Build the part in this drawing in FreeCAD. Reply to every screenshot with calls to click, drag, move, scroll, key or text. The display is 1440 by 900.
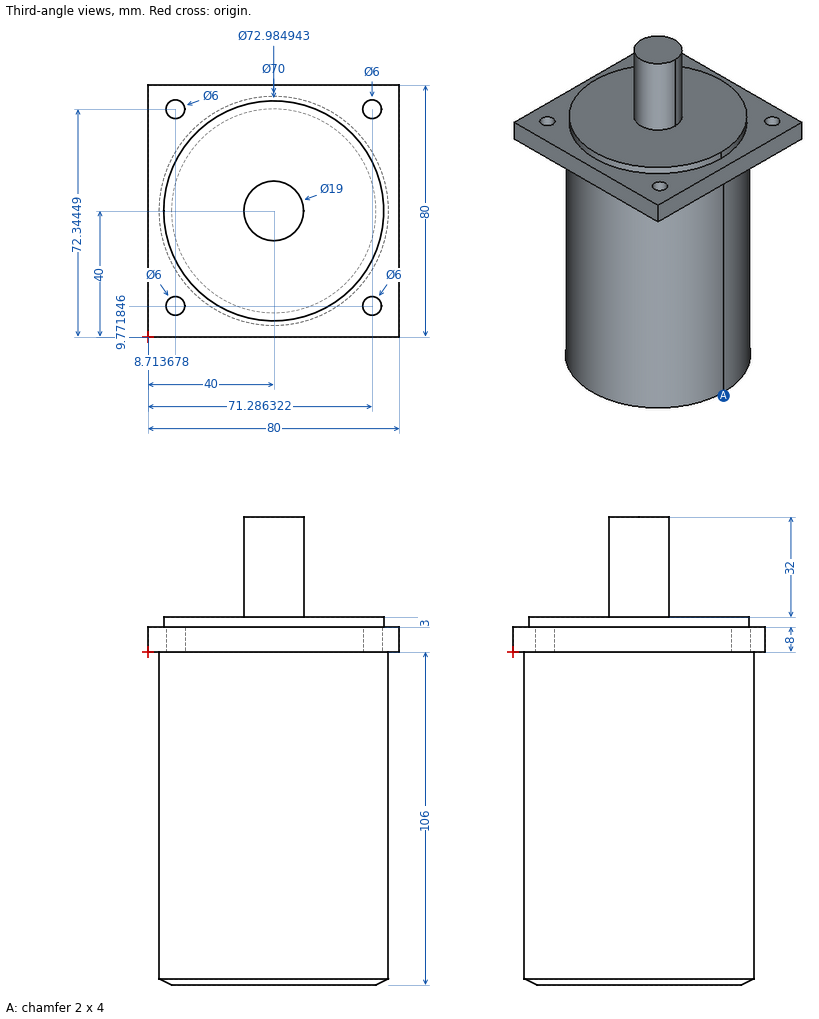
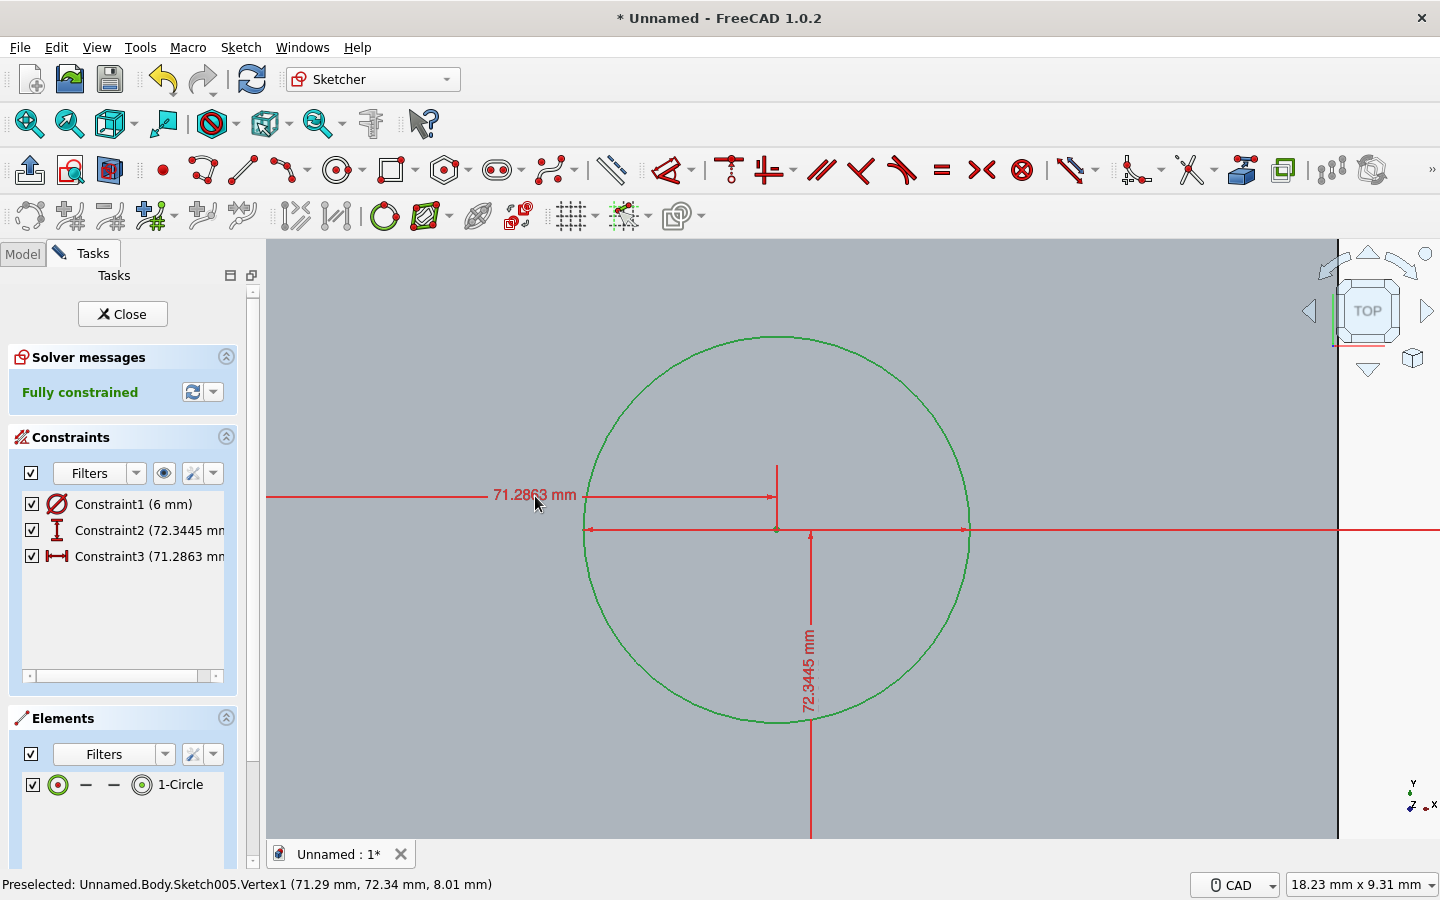
click(123, 314)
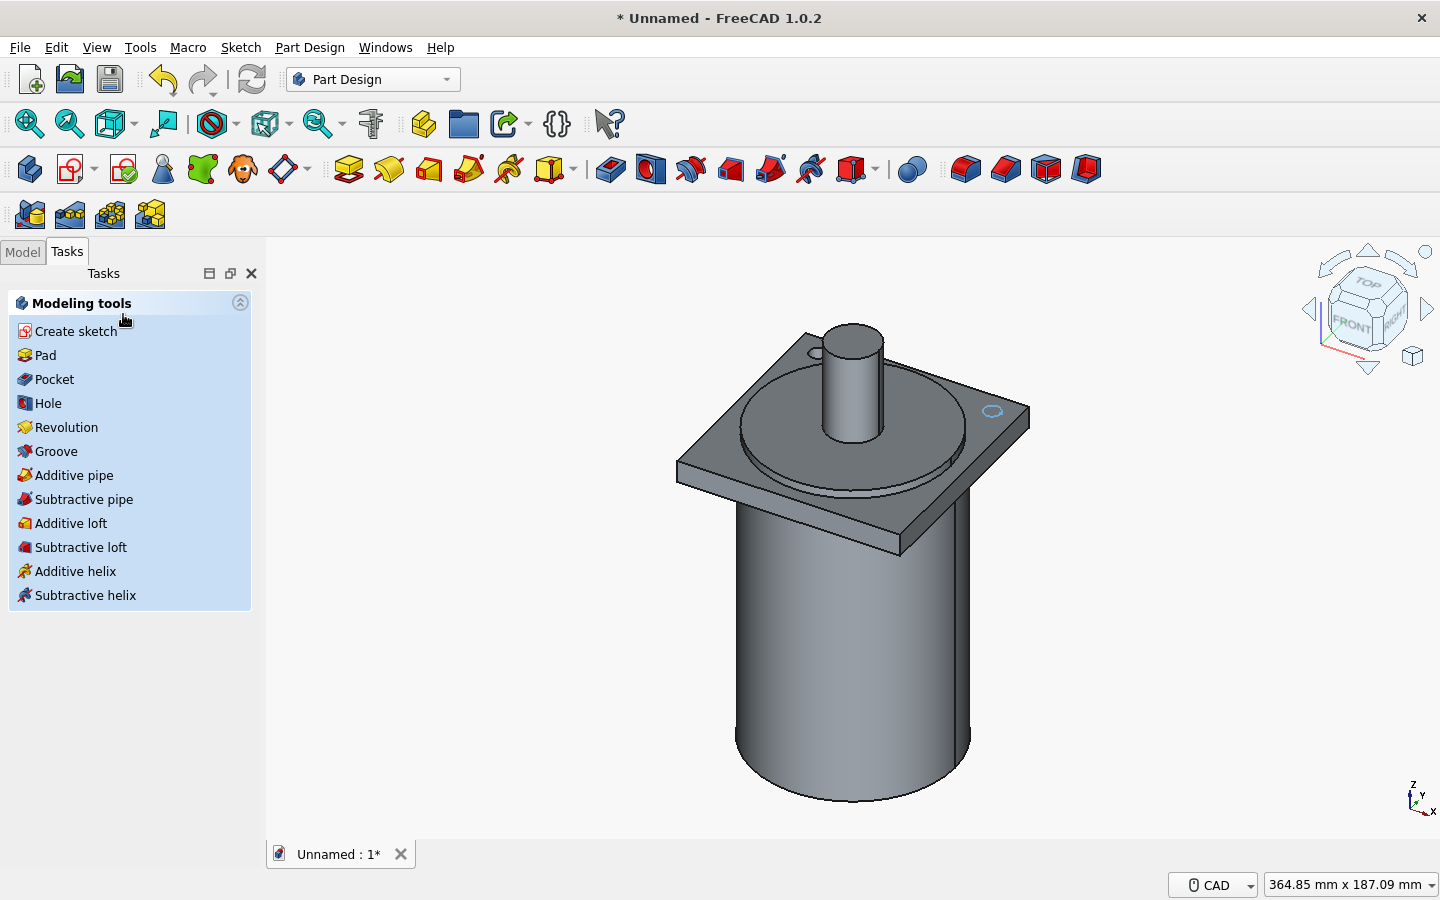
click(612, 170)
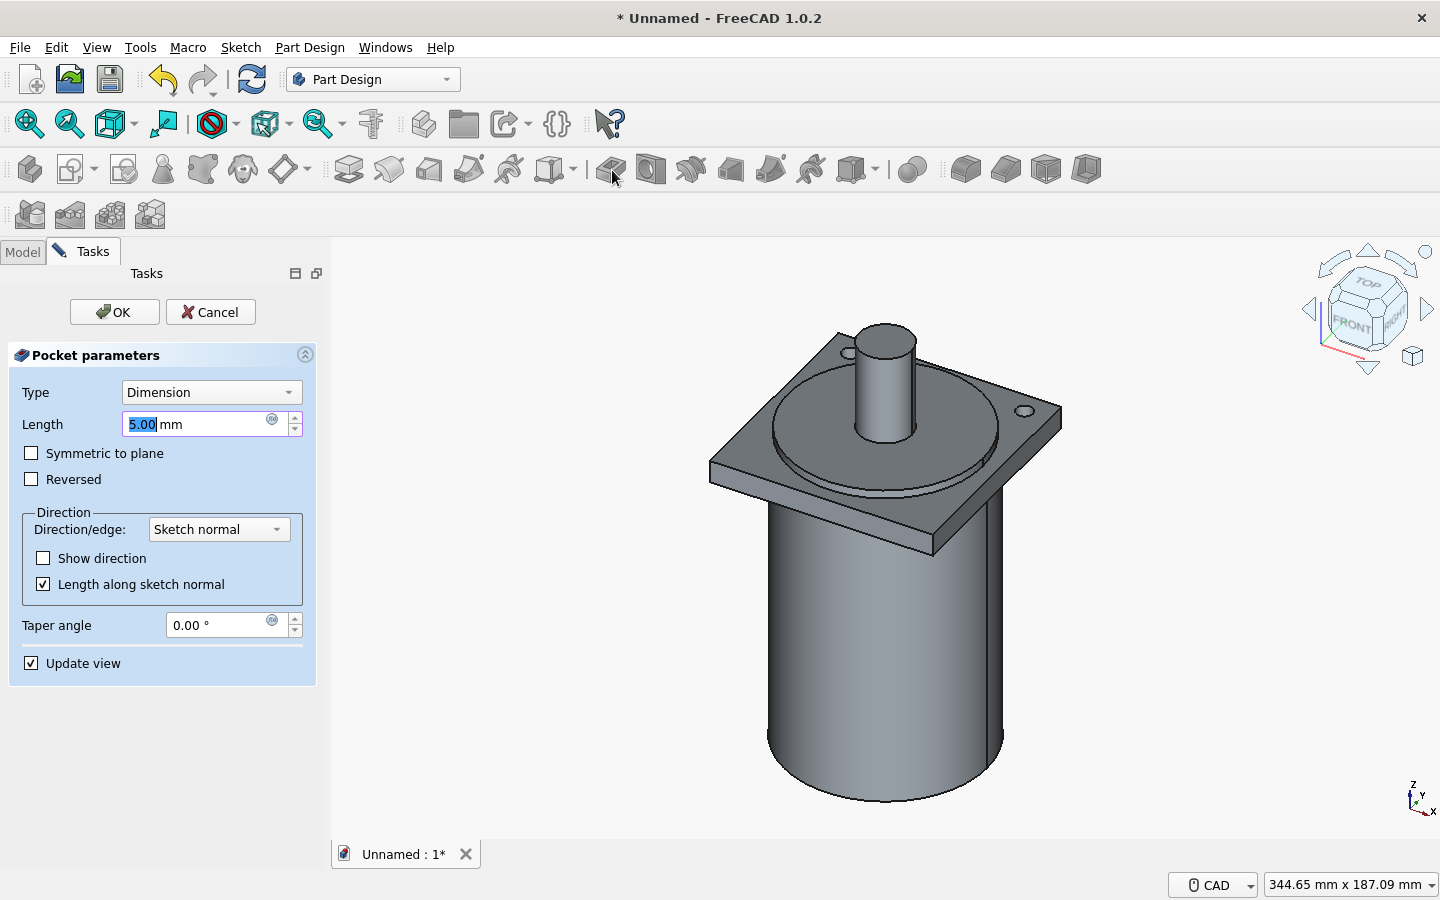
click(212, 392)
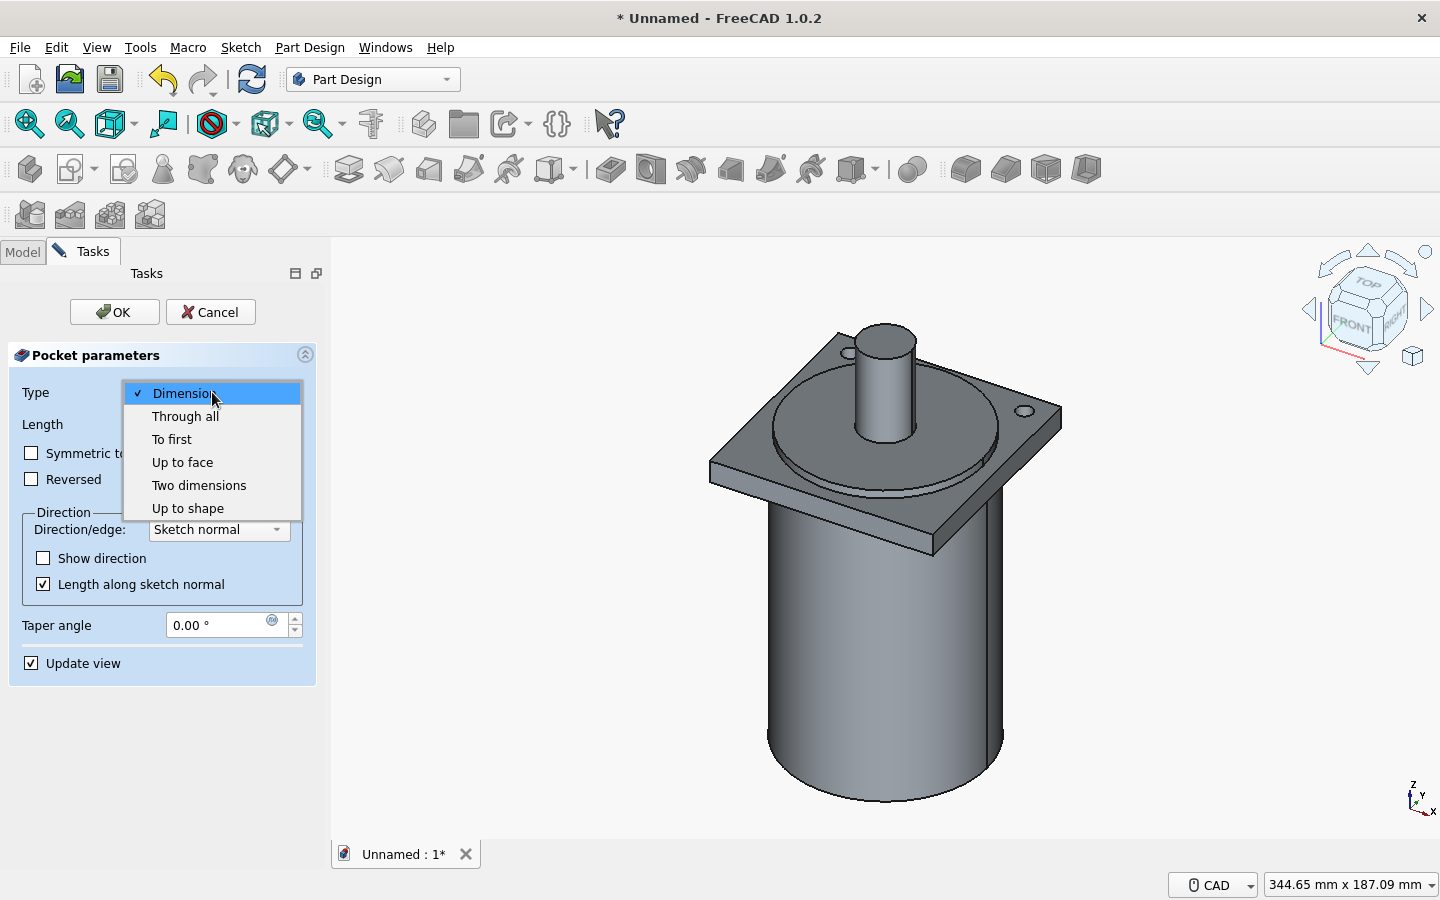
click(212, 440)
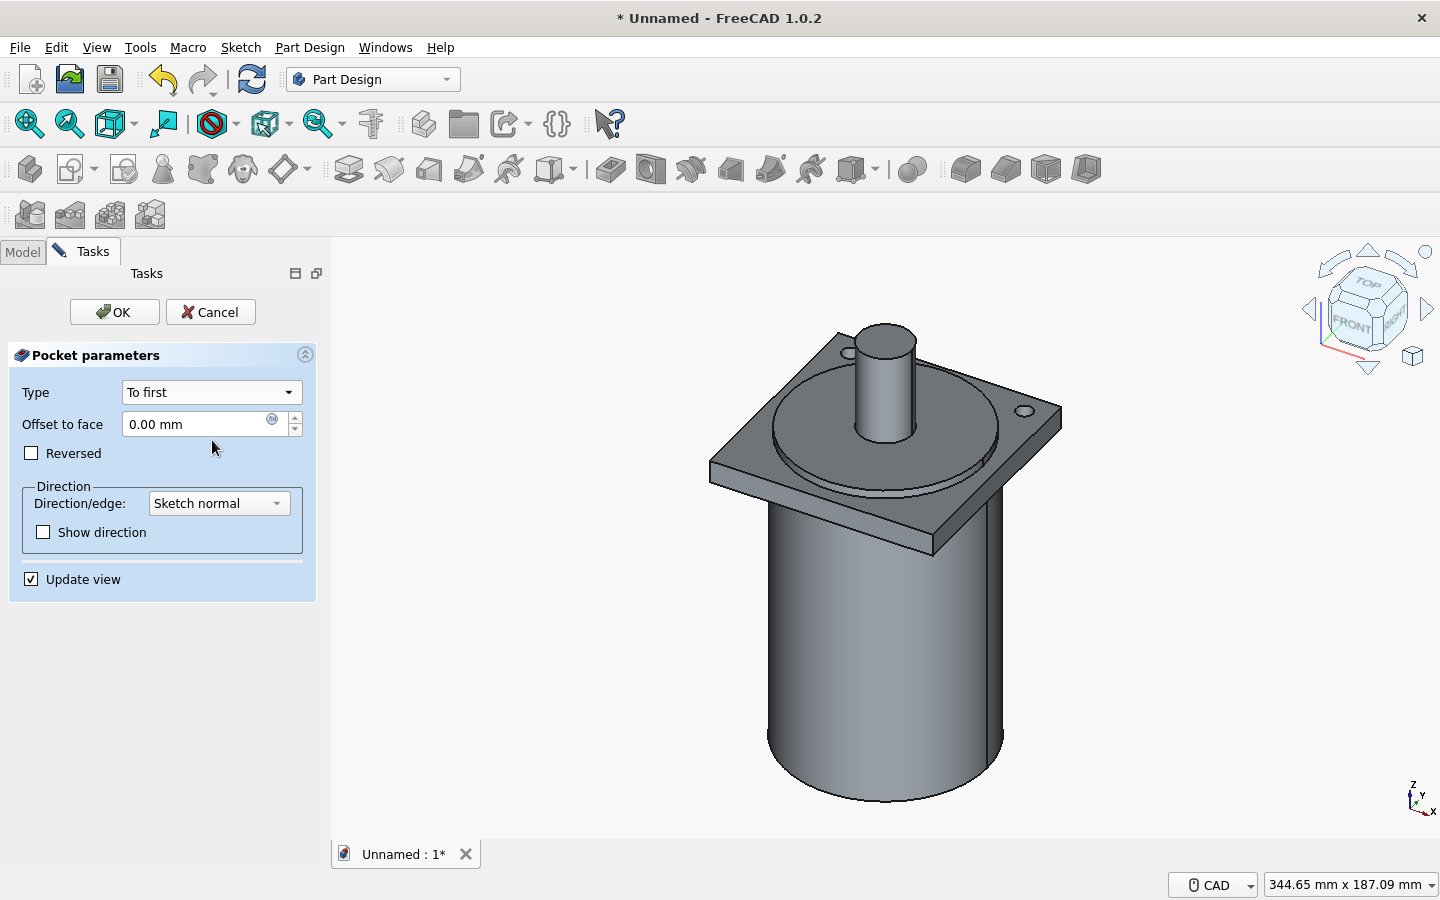
click(115, 312)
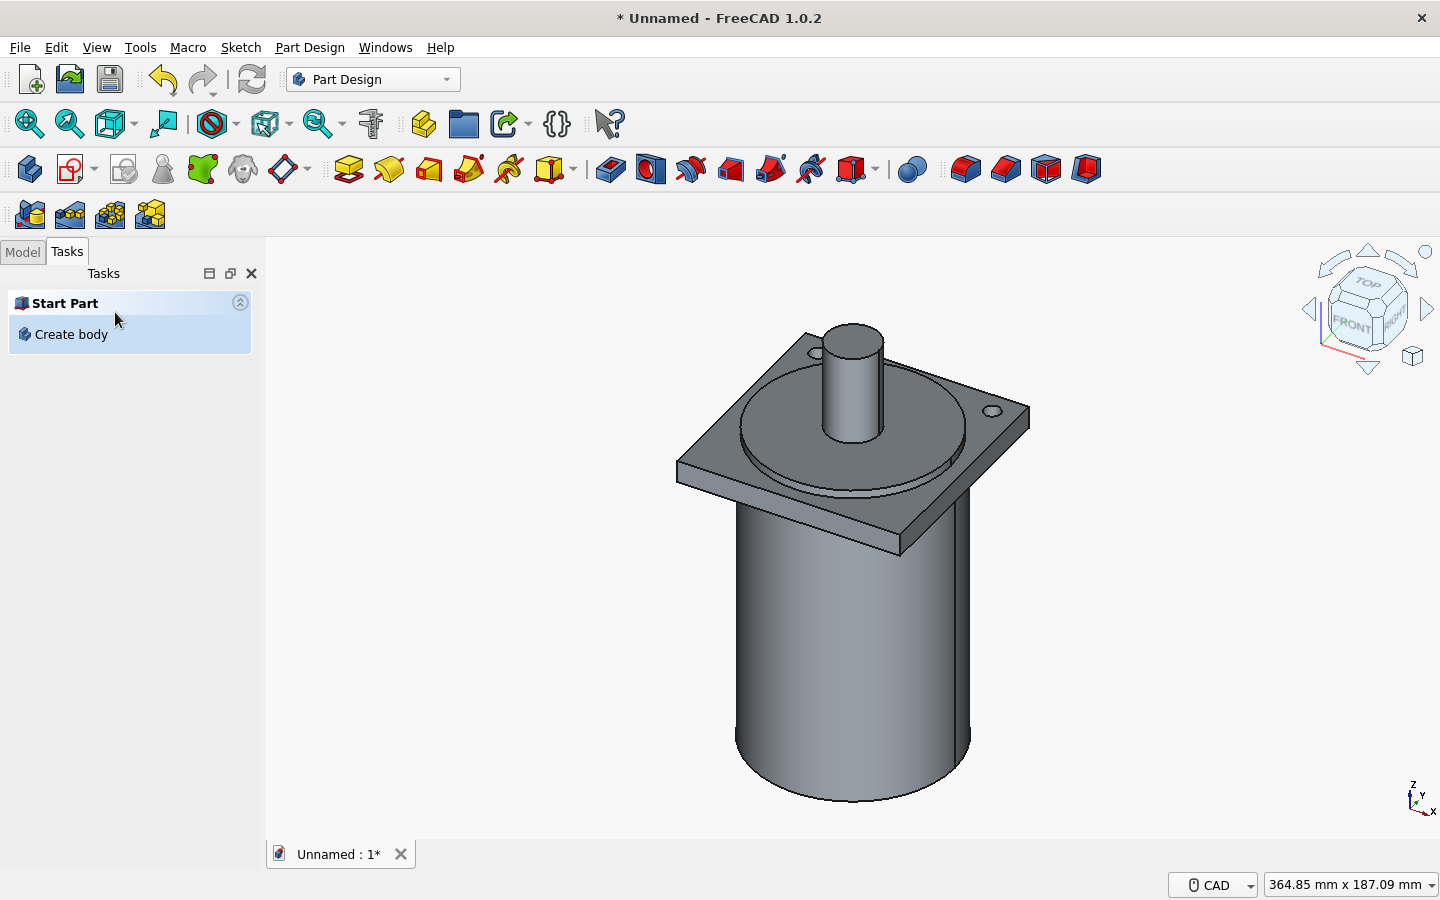
click(862, 509)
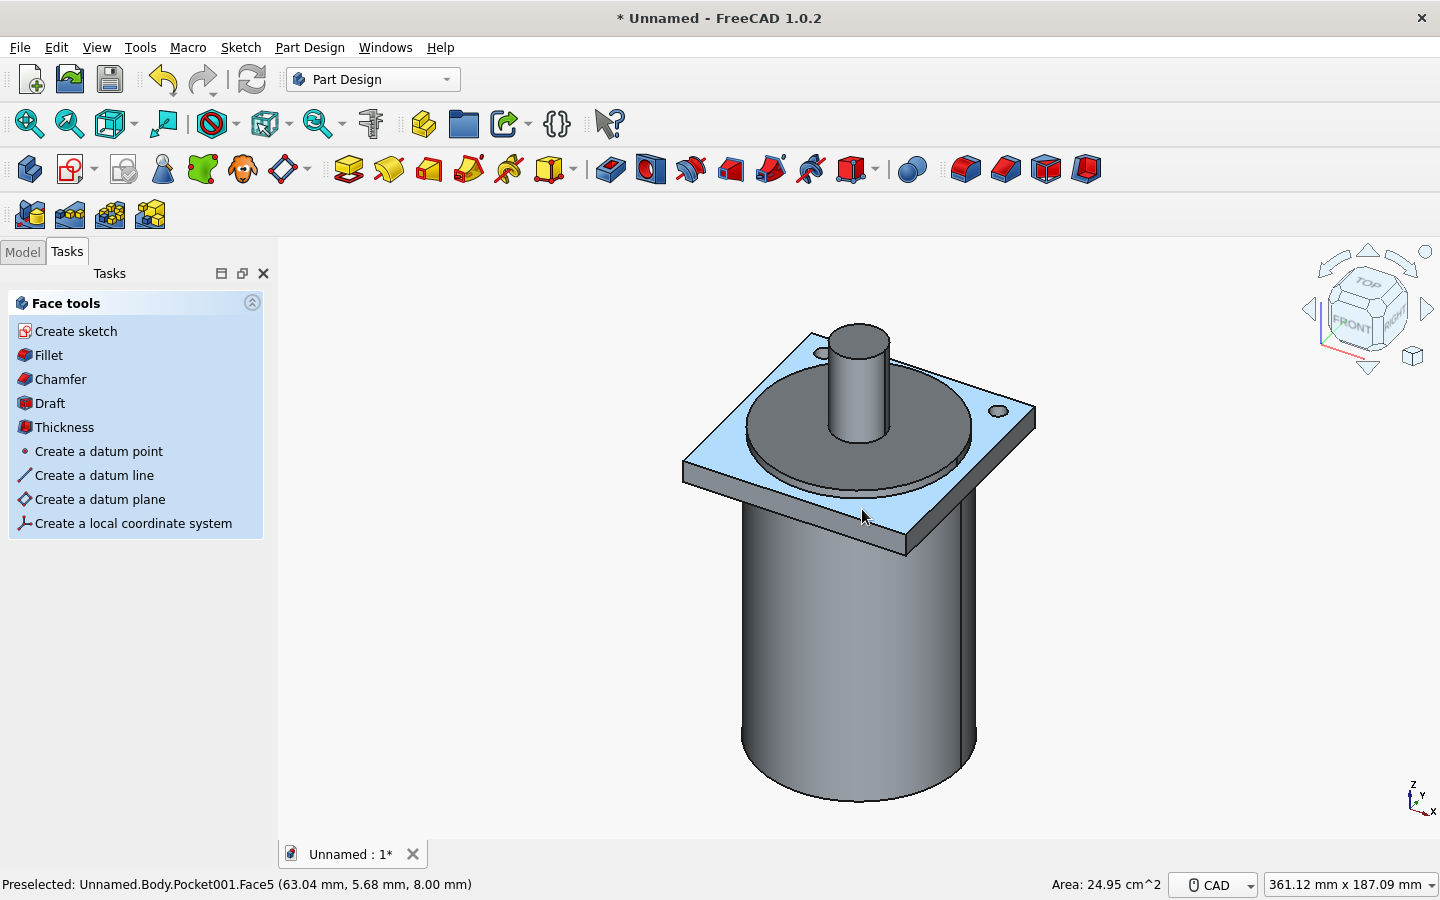
click(70, 170)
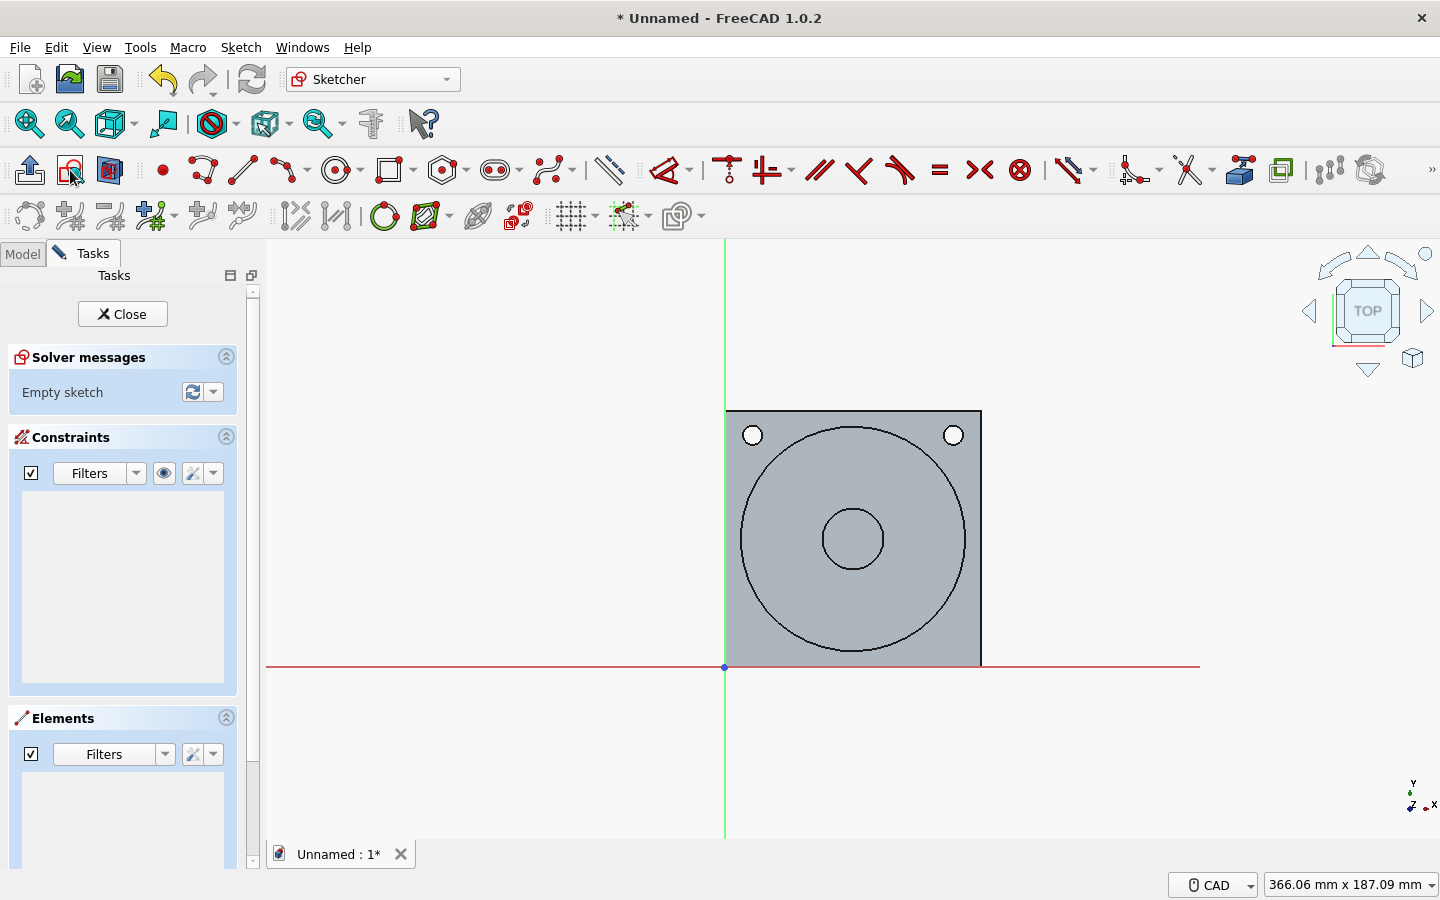
click(110, 170)